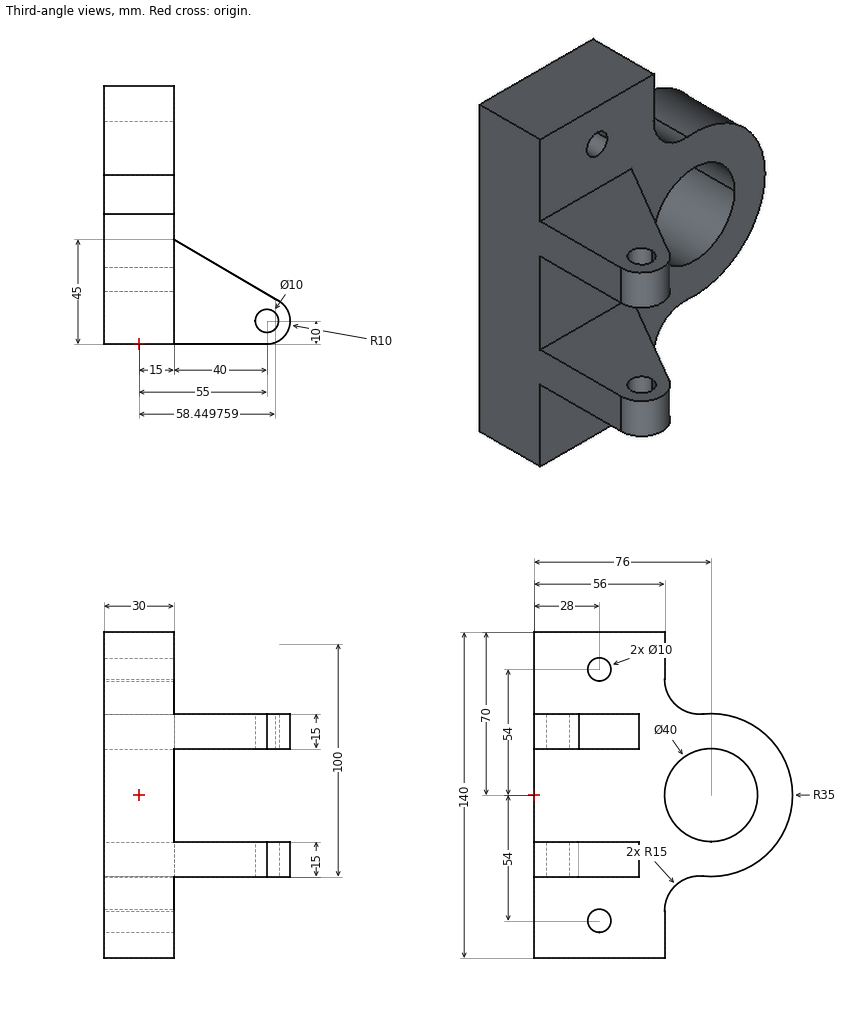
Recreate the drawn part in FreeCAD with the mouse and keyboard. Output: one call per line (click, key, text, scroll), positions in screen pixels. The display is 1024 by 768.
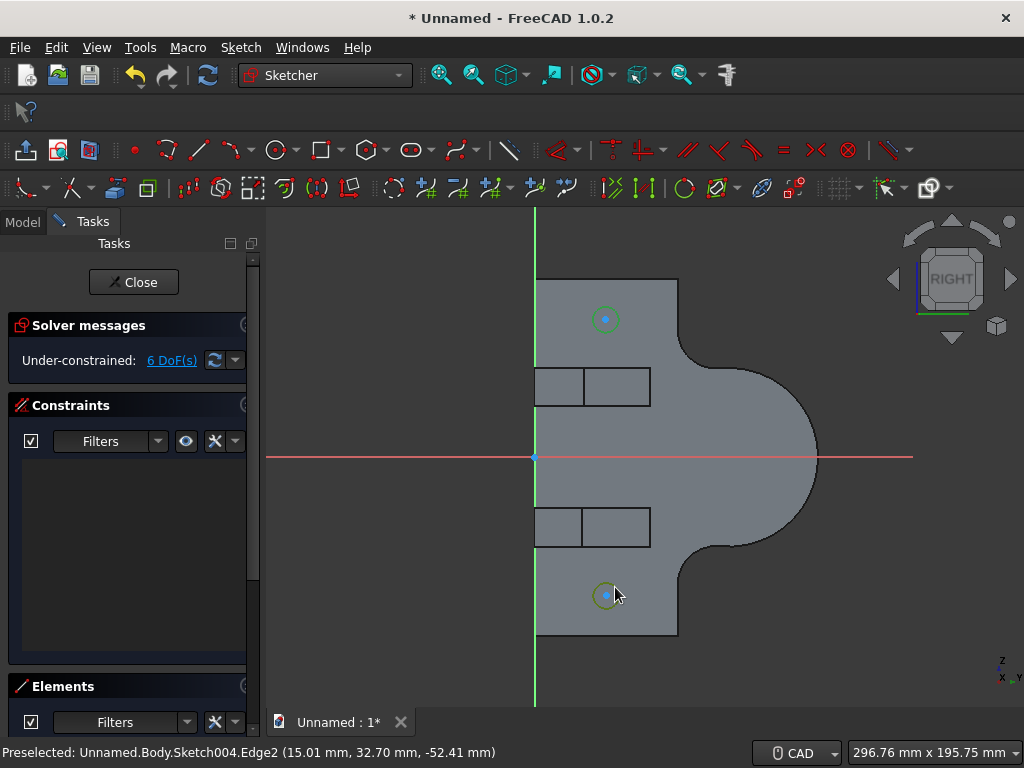
click(784, 150)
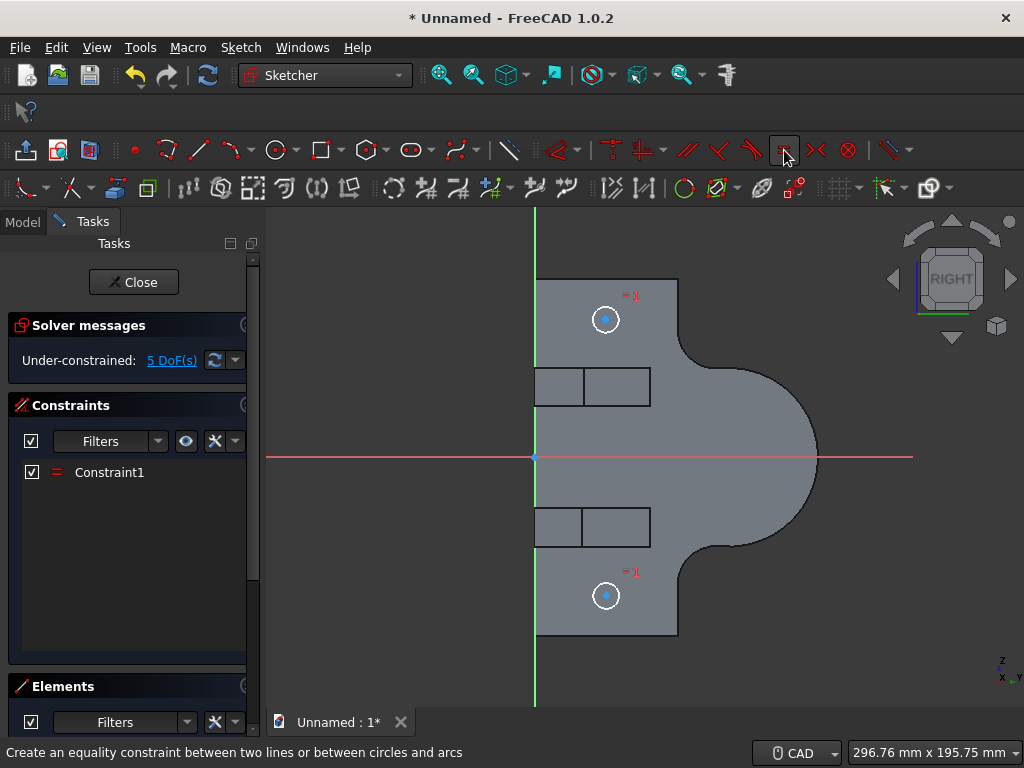
click(606, 320)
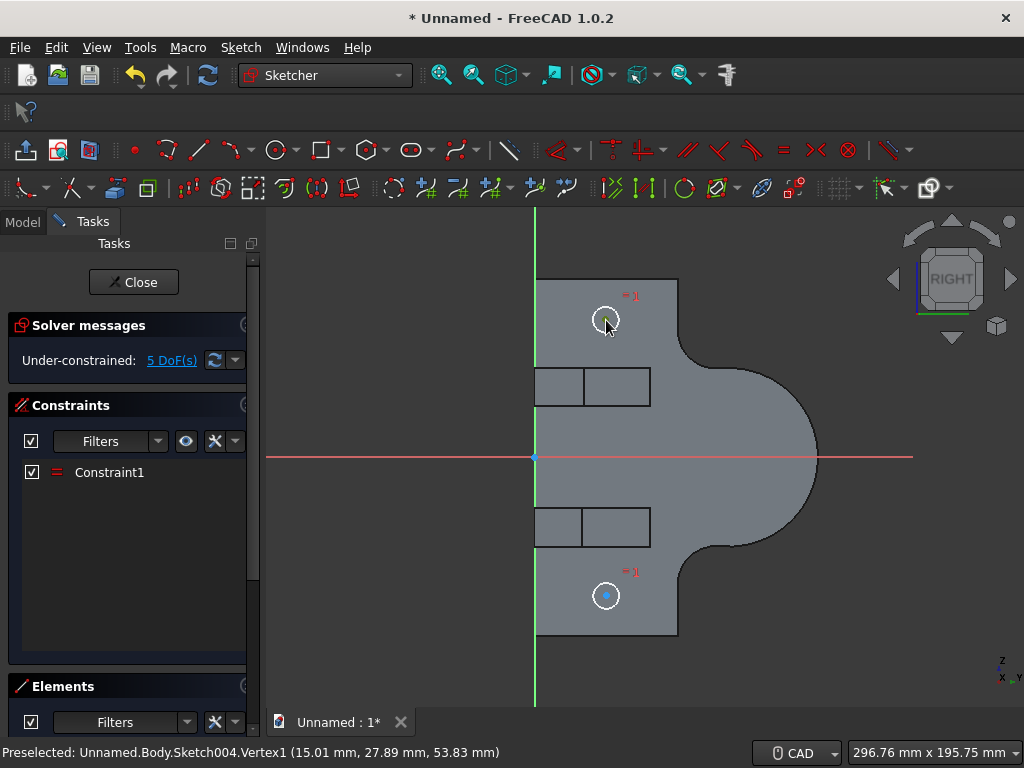
click(606, 596)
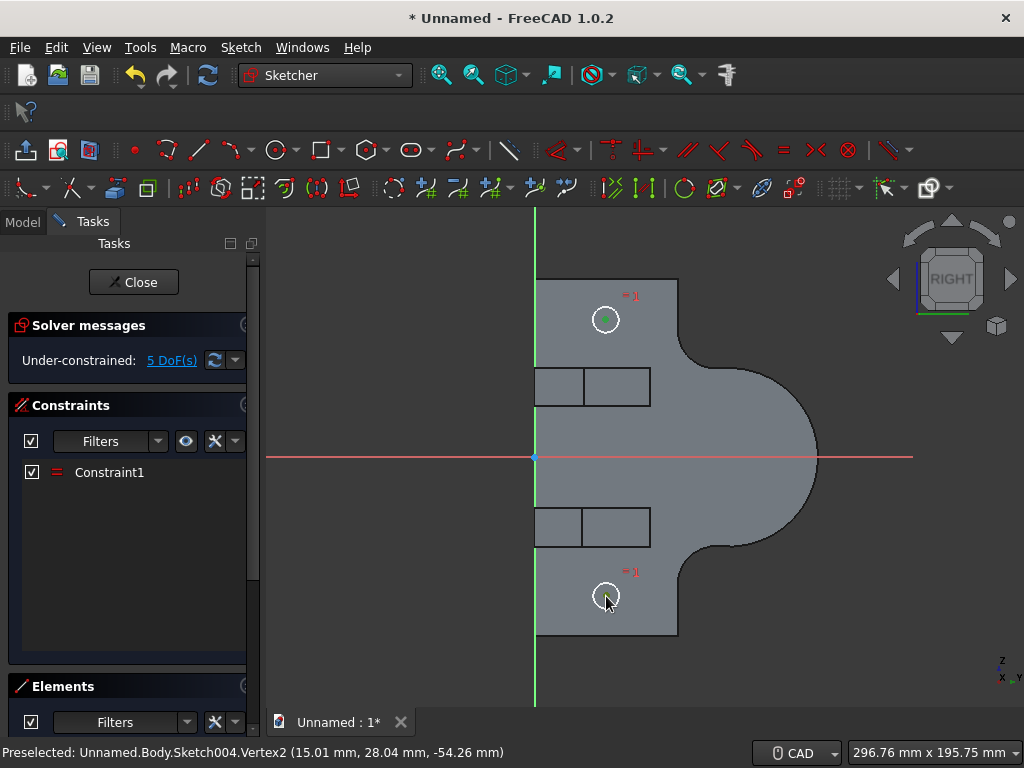
key(v)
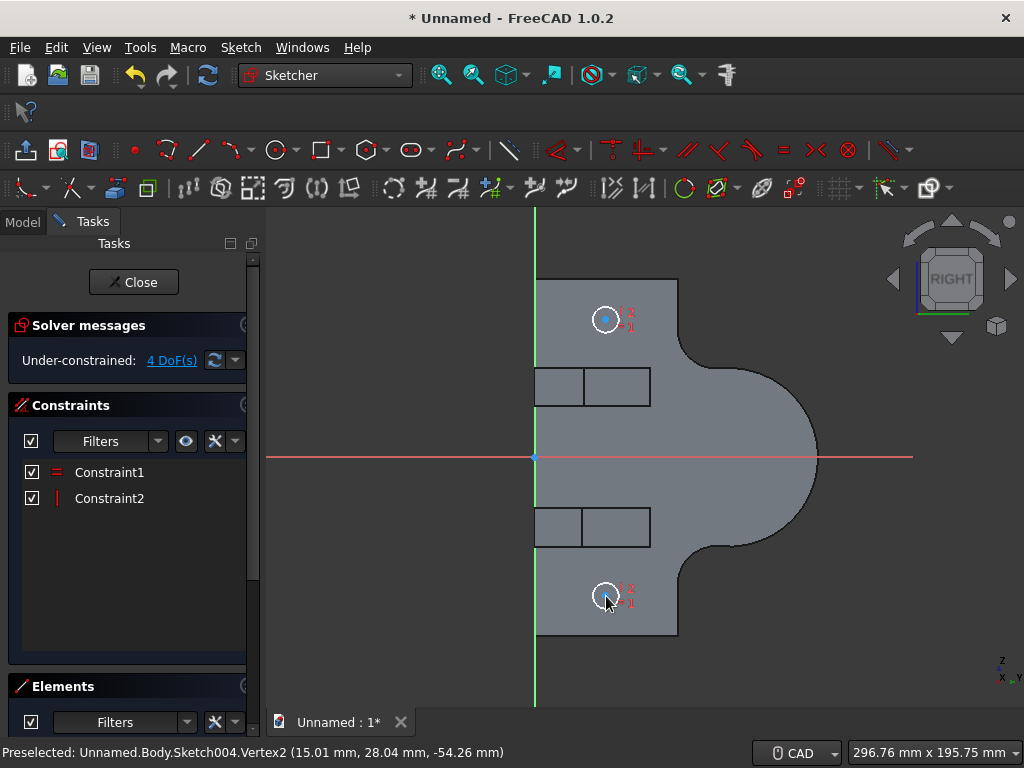
key(d)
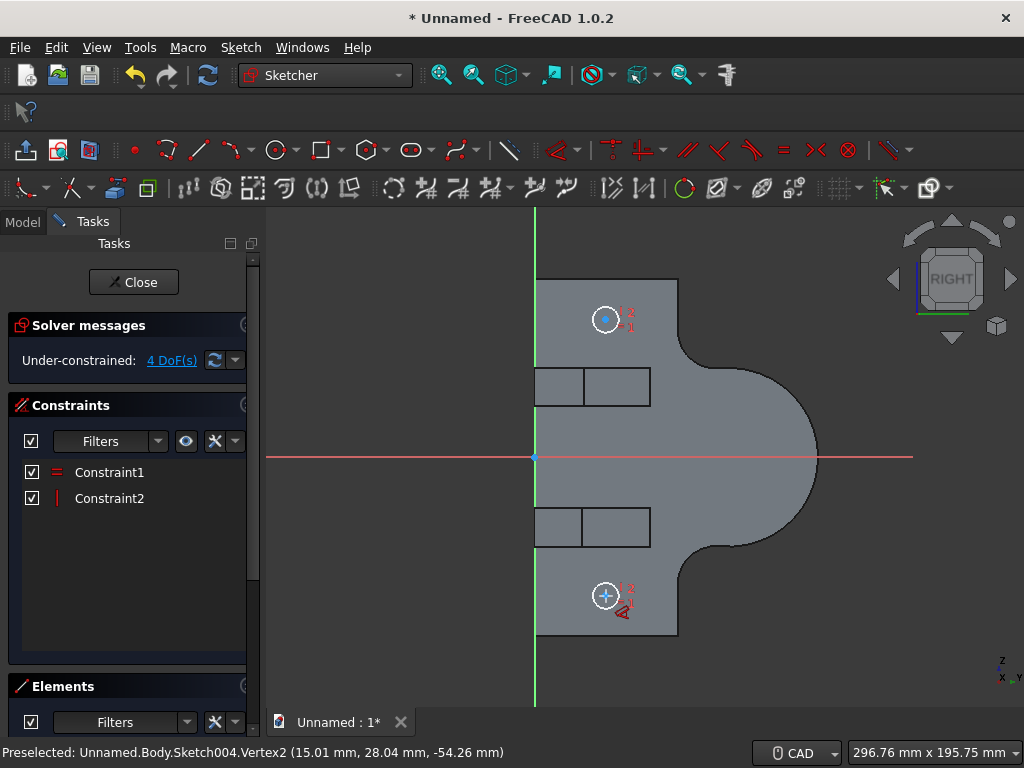
scroll(615, 311, up, 3)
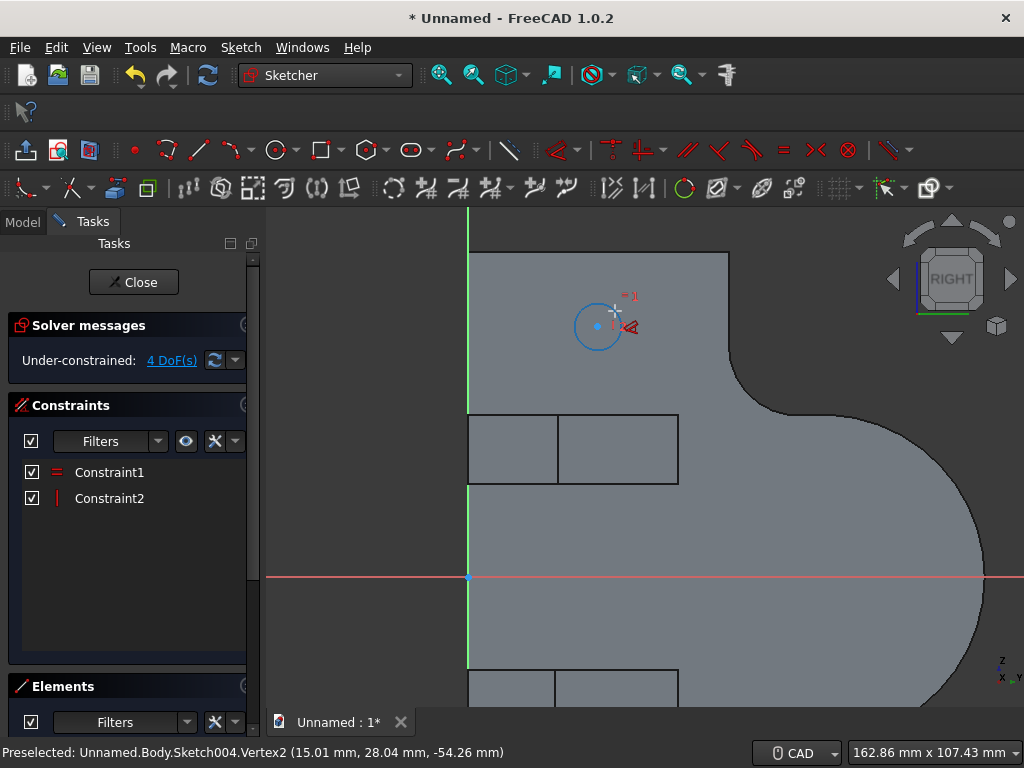
click(614, 310)
click(636, 287)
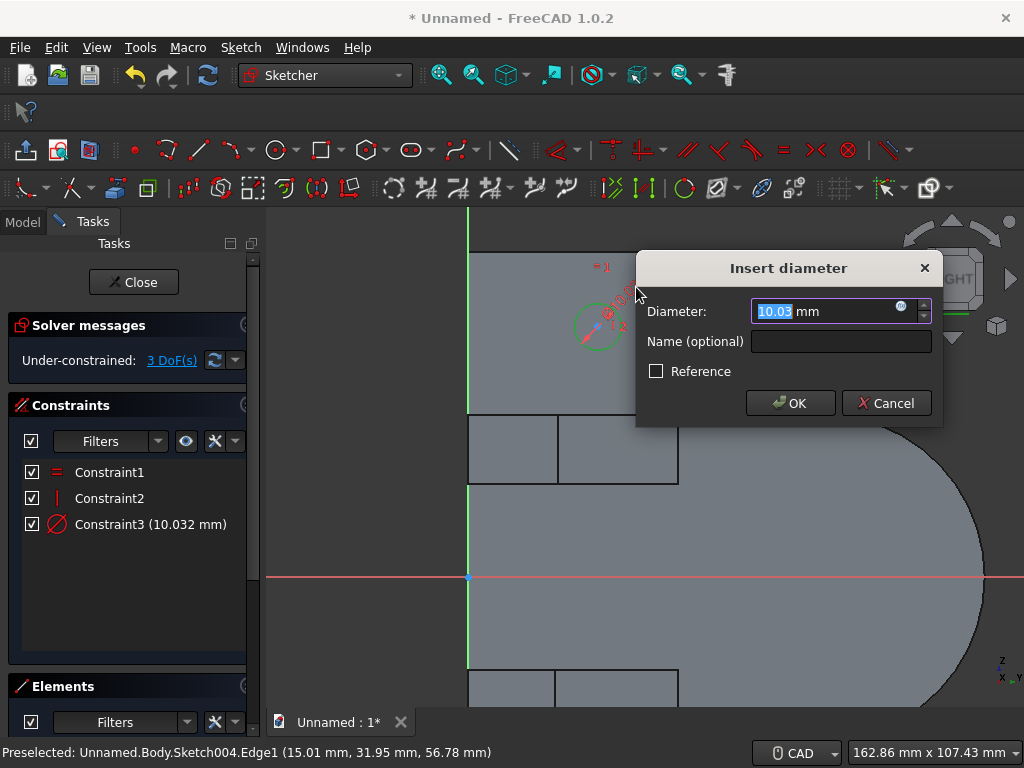
text(10)
key(Return)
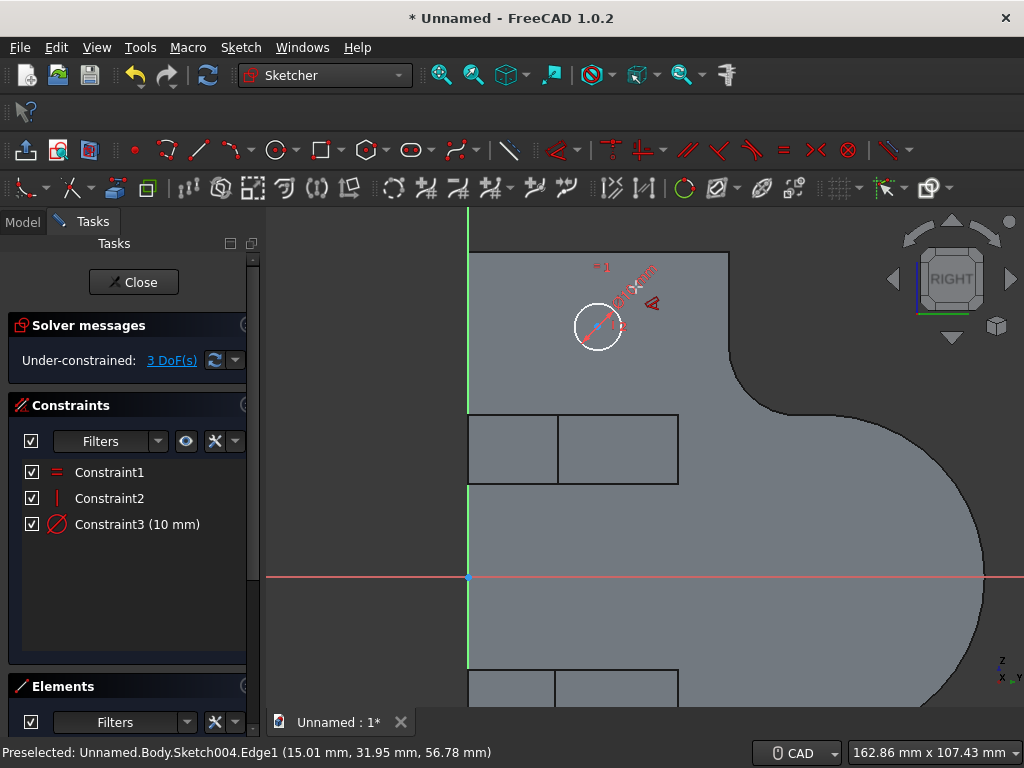
click(598, 327)
click(533, 293)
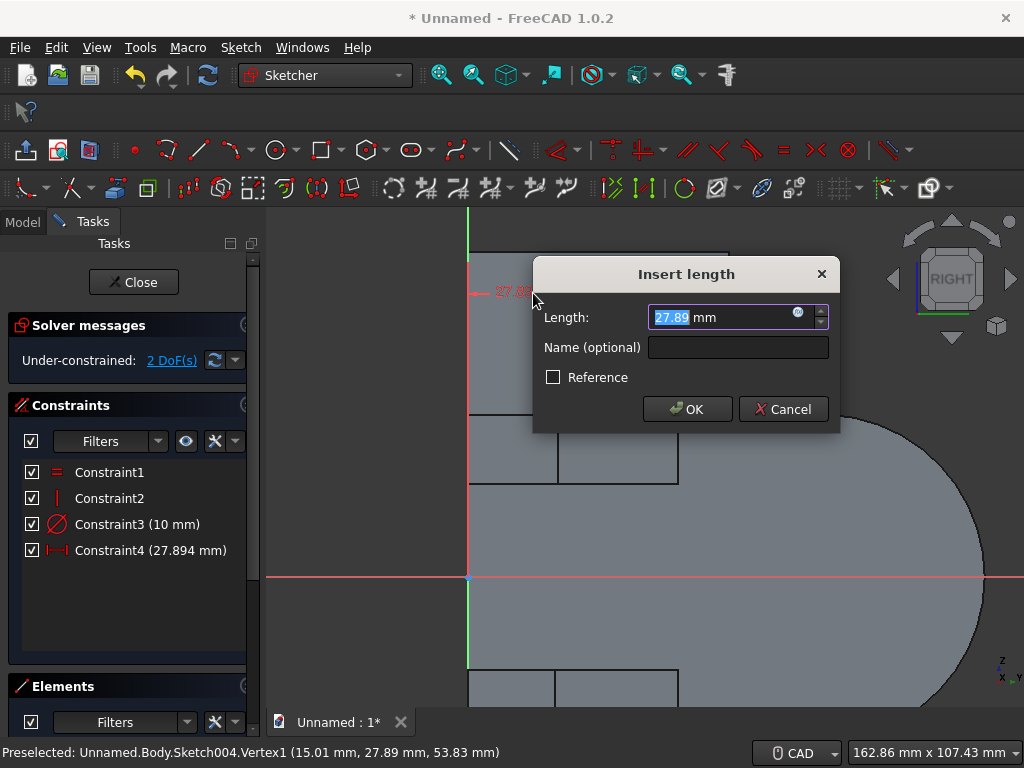
text(28)
key(Return)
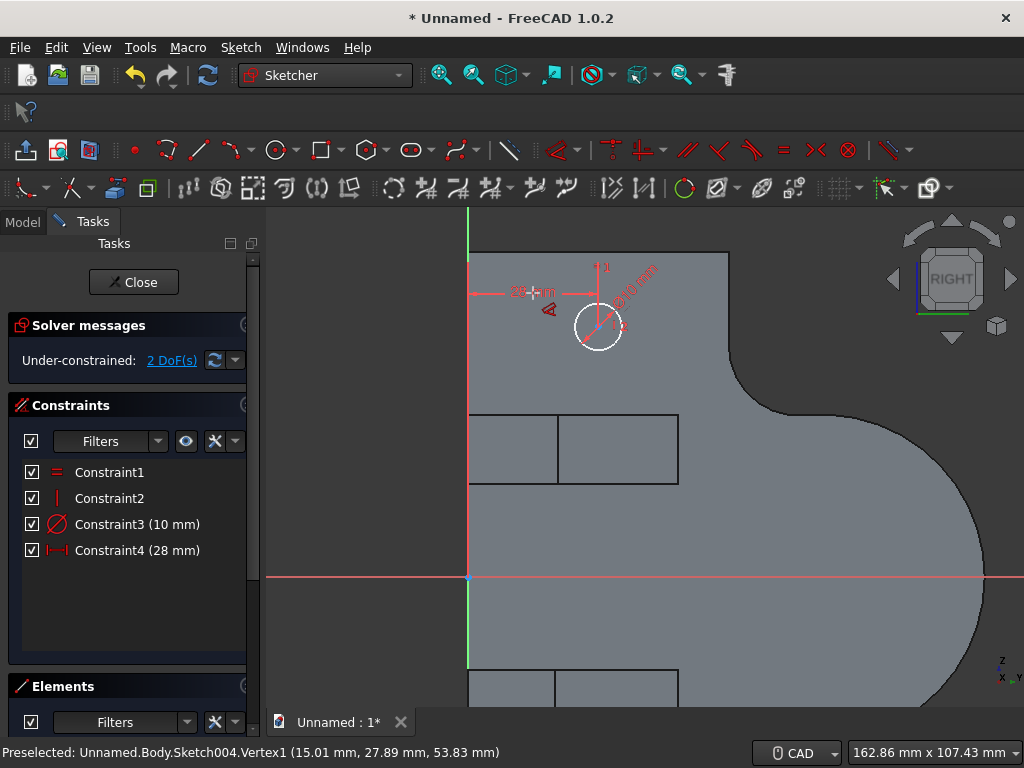
click(598, 327)
click(434, 452)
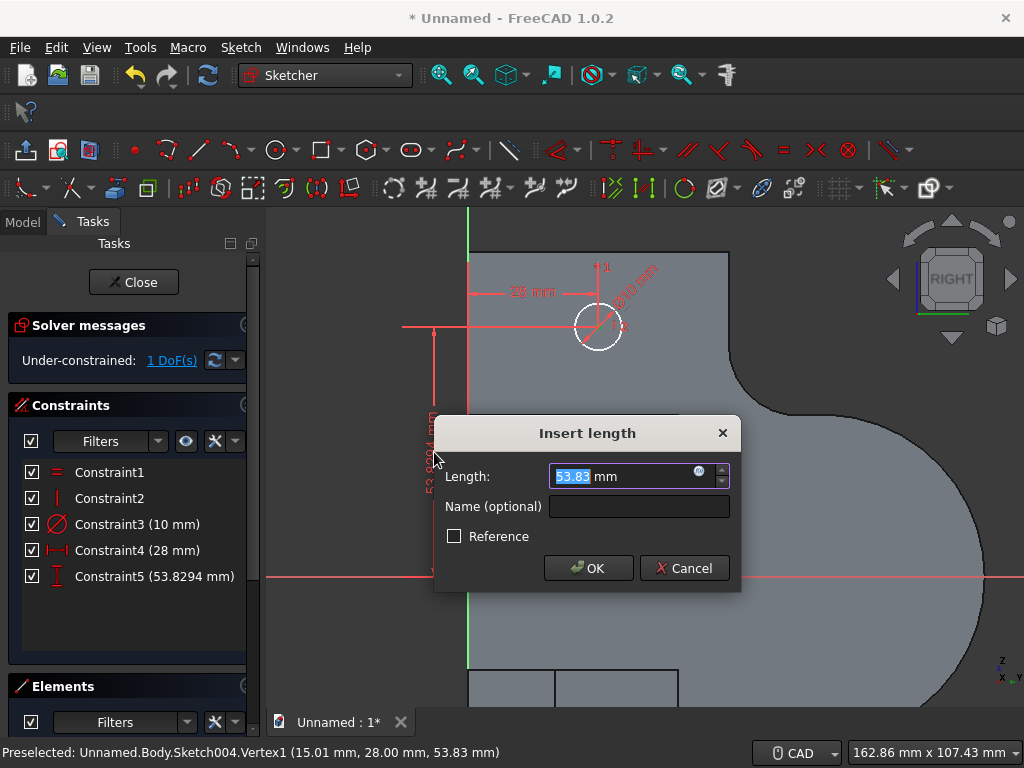
text(54)
key(Return)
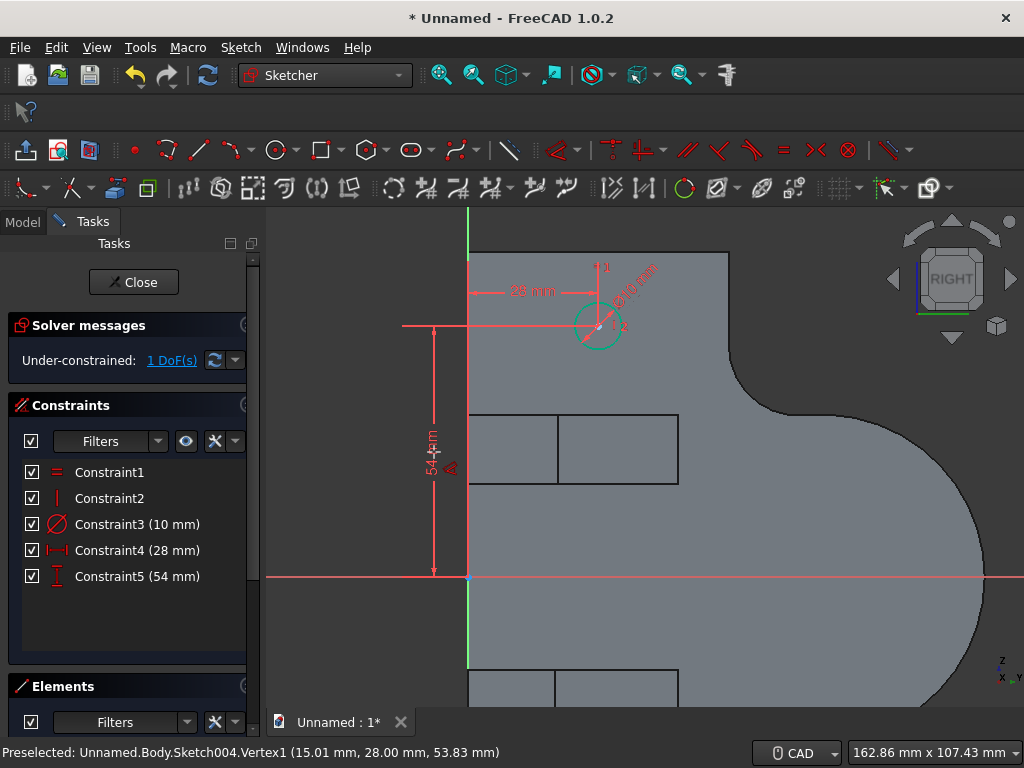
scroll(615, 311, down, 3)